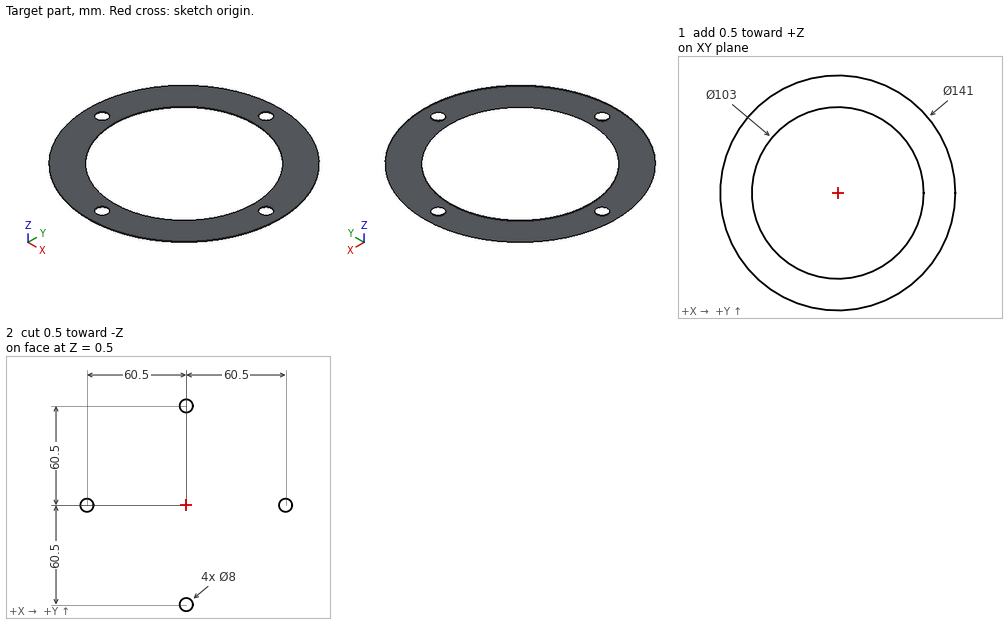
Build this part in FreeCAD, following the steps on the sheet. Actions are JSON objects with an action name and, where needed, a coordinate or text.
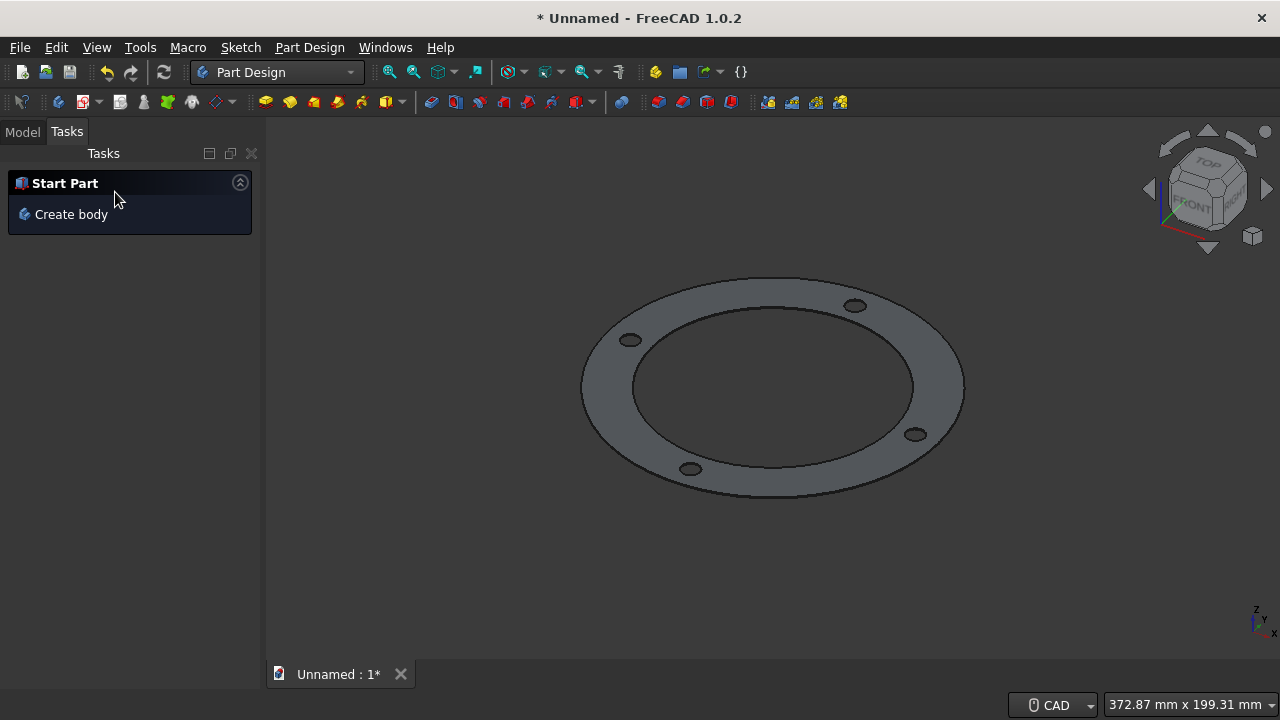
{"action": "key", "text": "0"}